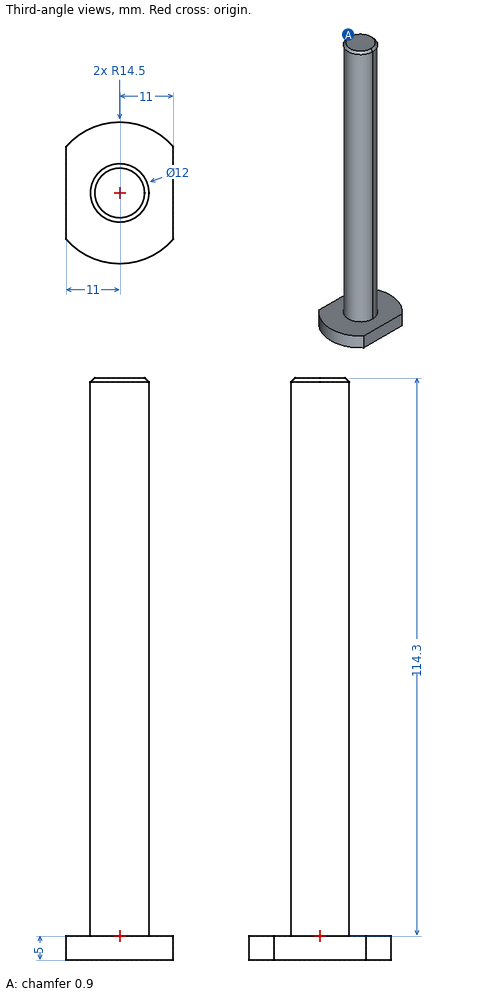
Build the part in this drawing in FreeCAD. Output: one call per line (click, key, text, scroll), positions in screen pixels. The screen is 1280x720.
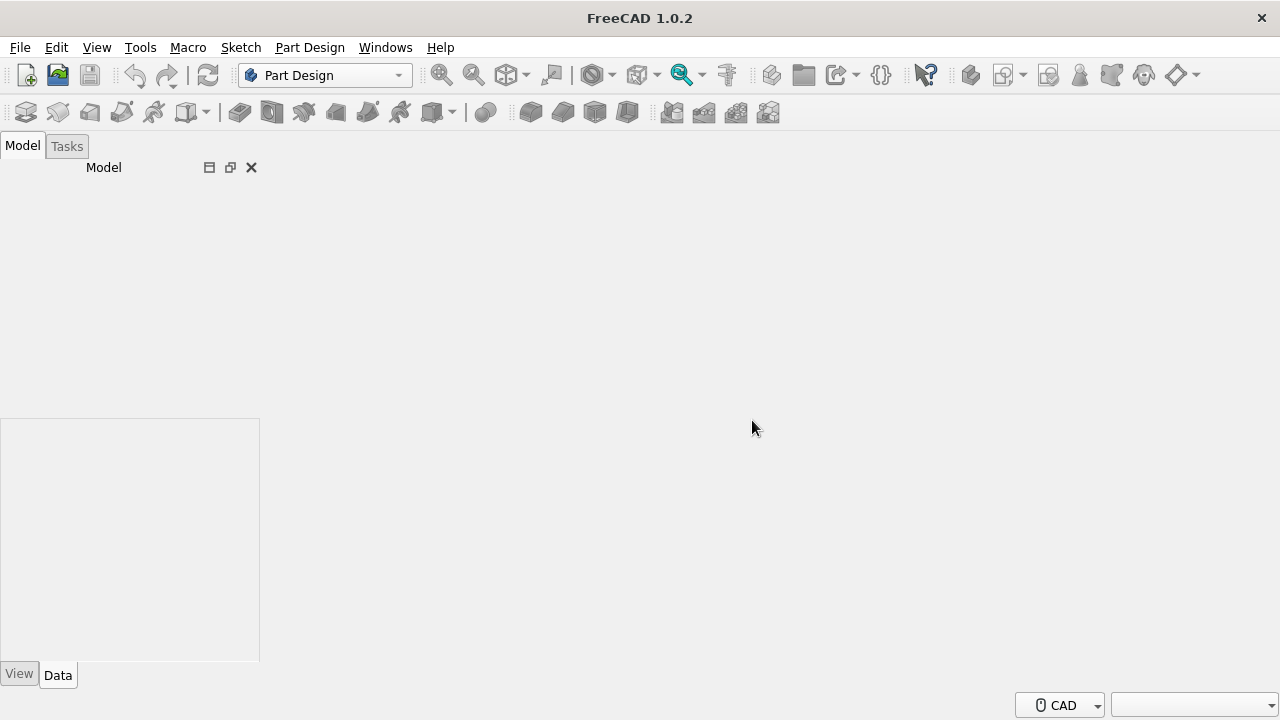
click(26, 76)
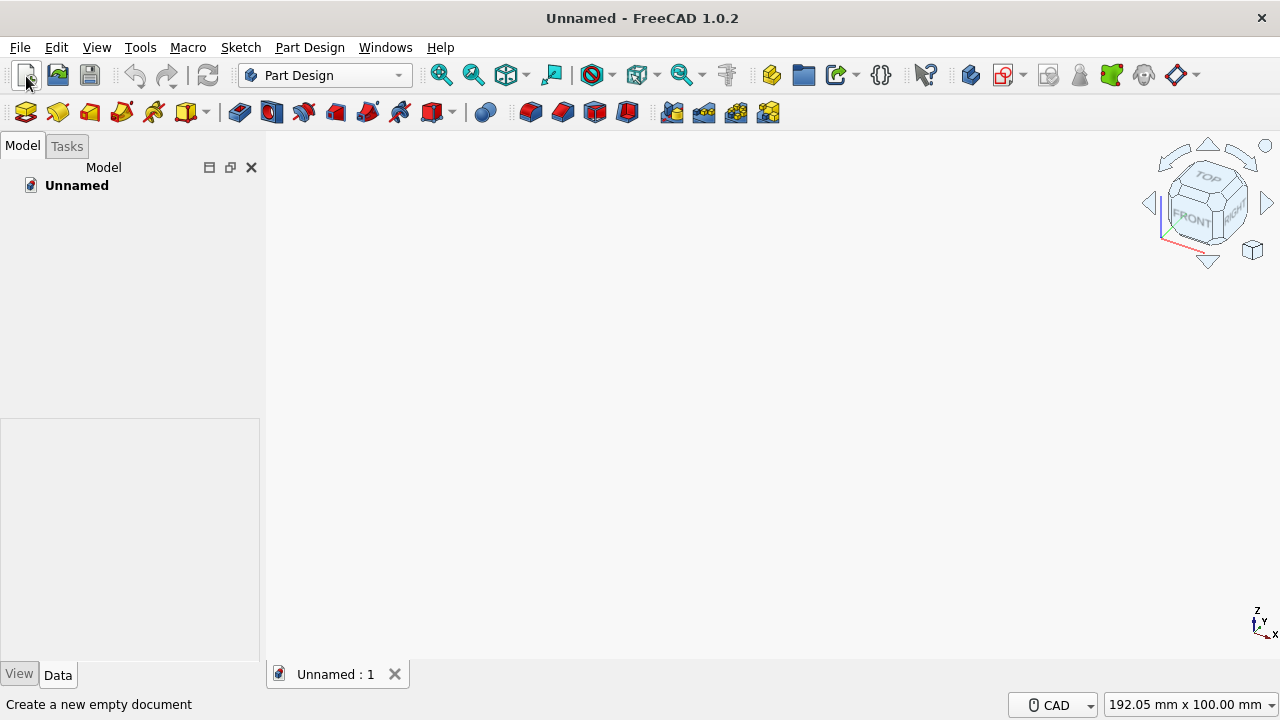
click(1004, 76)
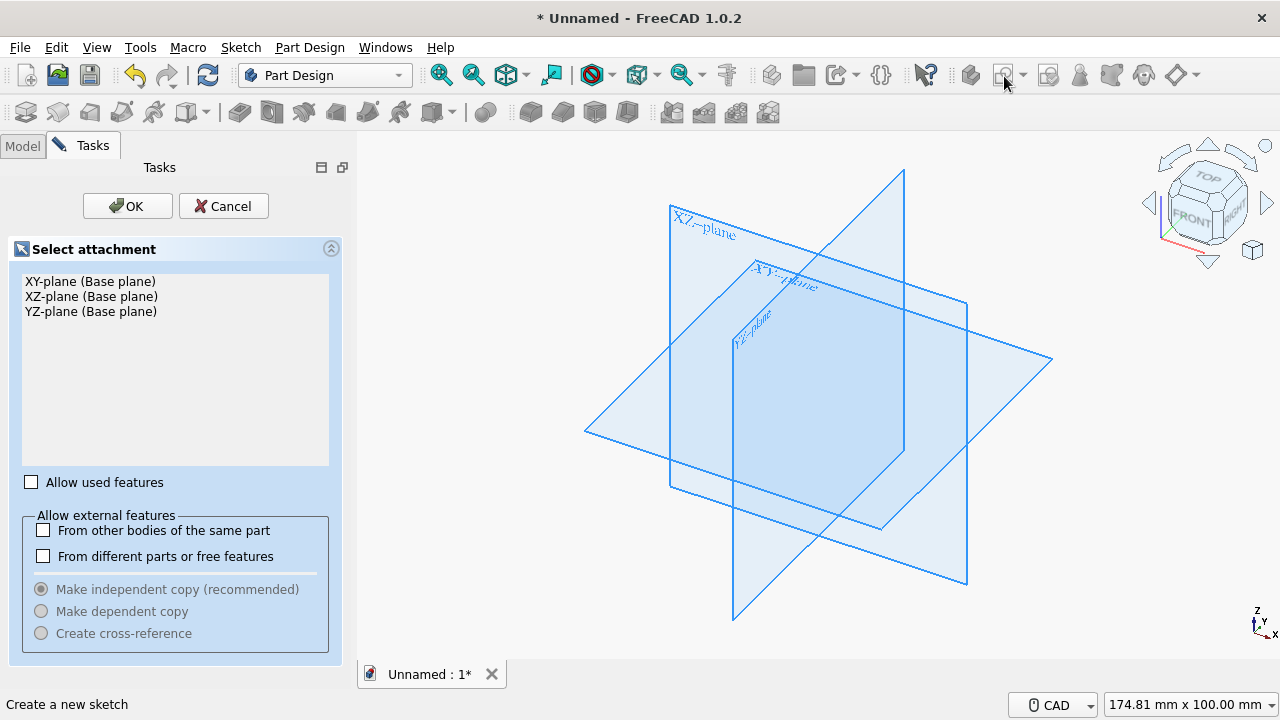
click(82, 282)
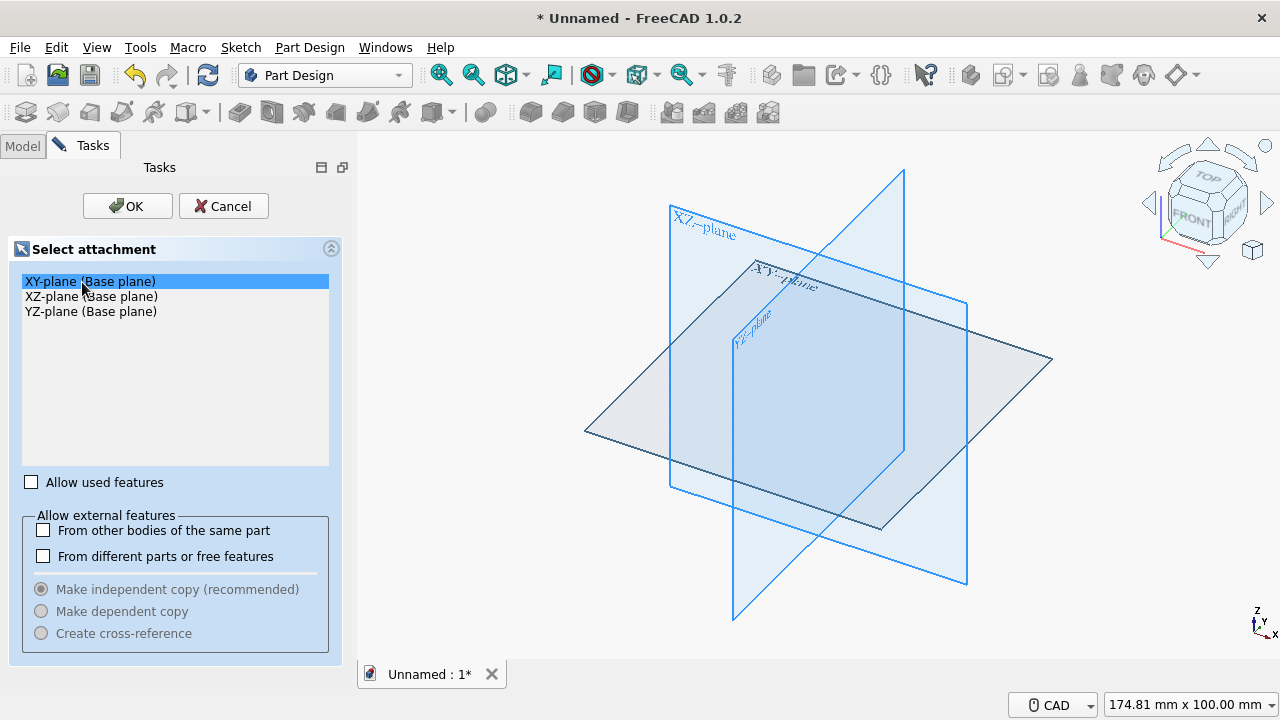
click(128, 206)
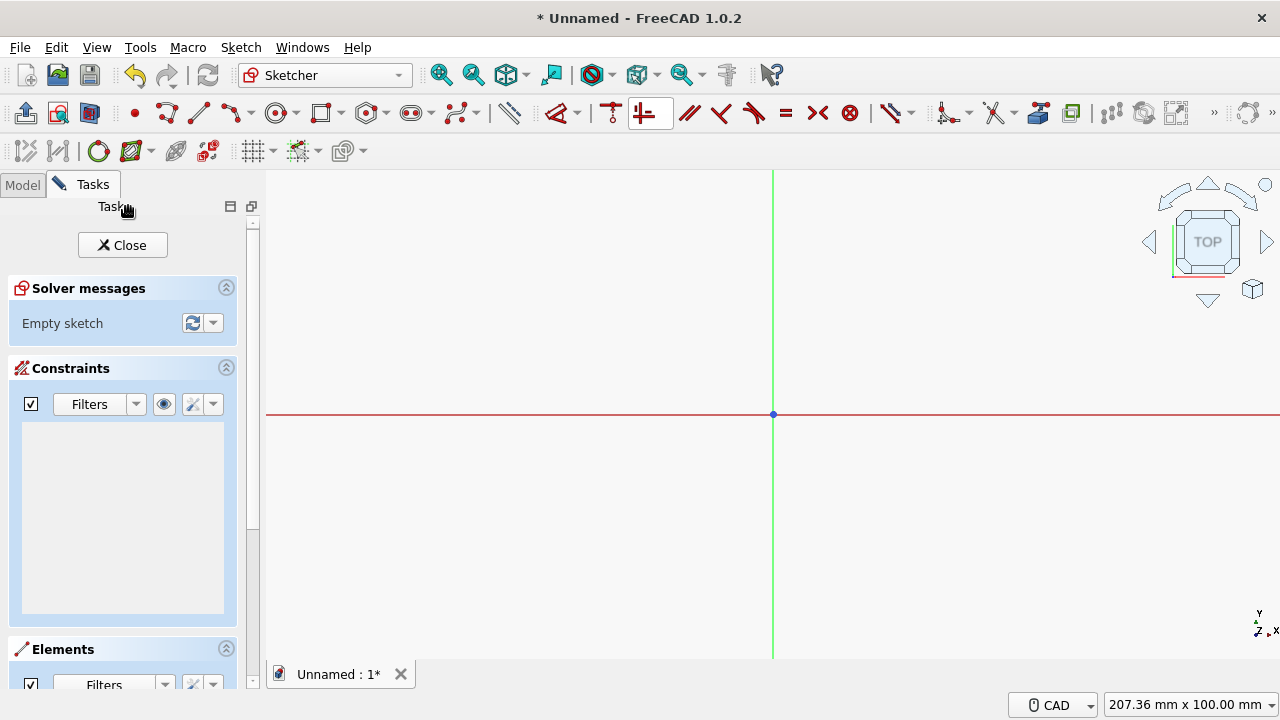
scroll(790, 414, up, 8)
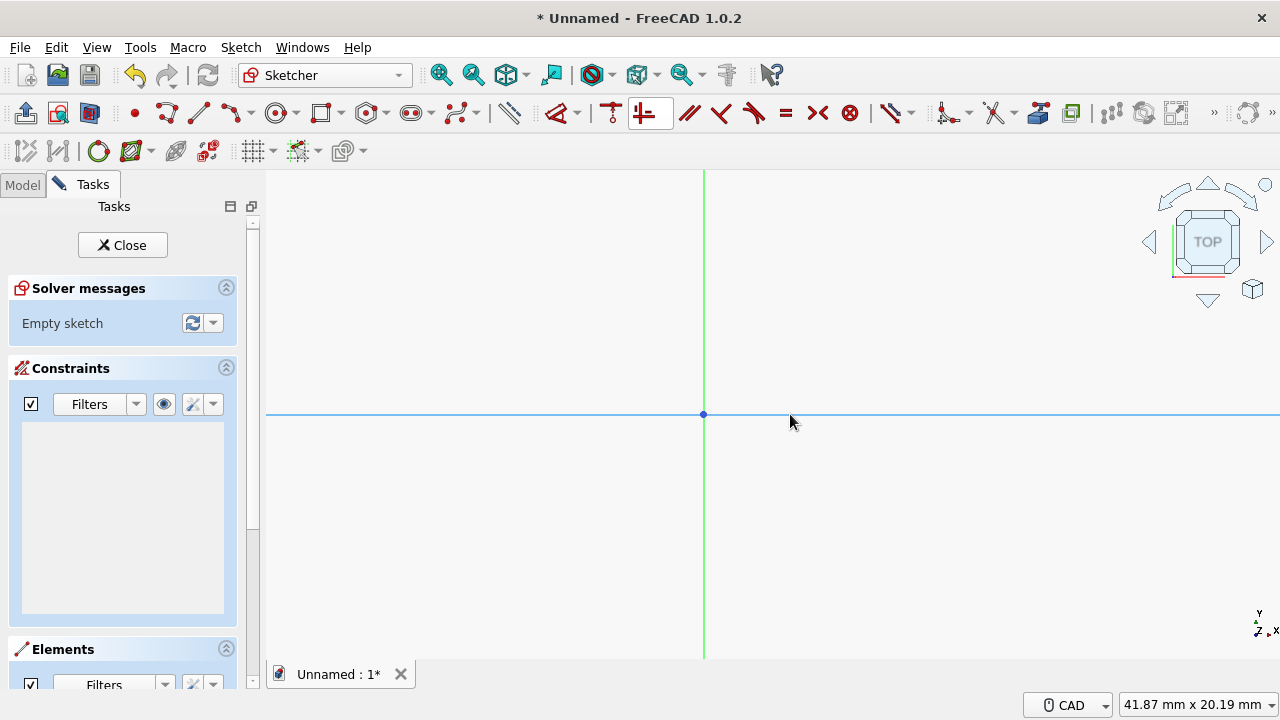
click(276, 114)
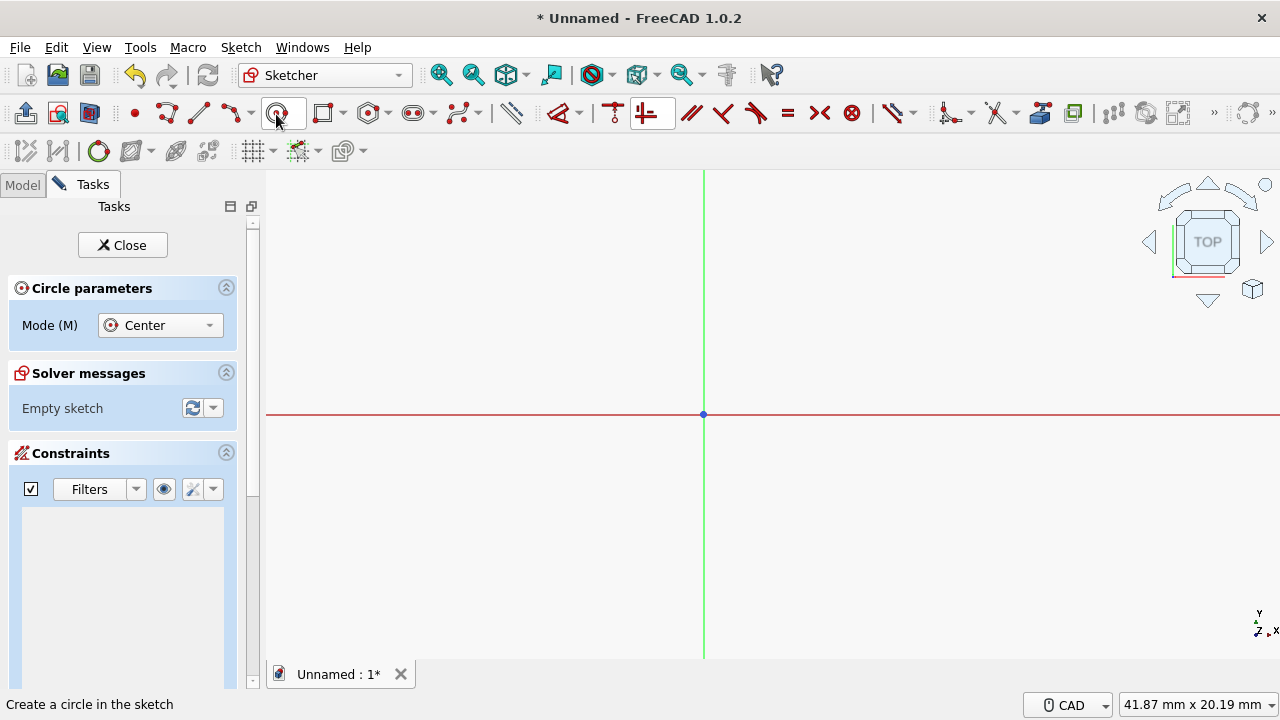
click(704, 414)
move(807, 312)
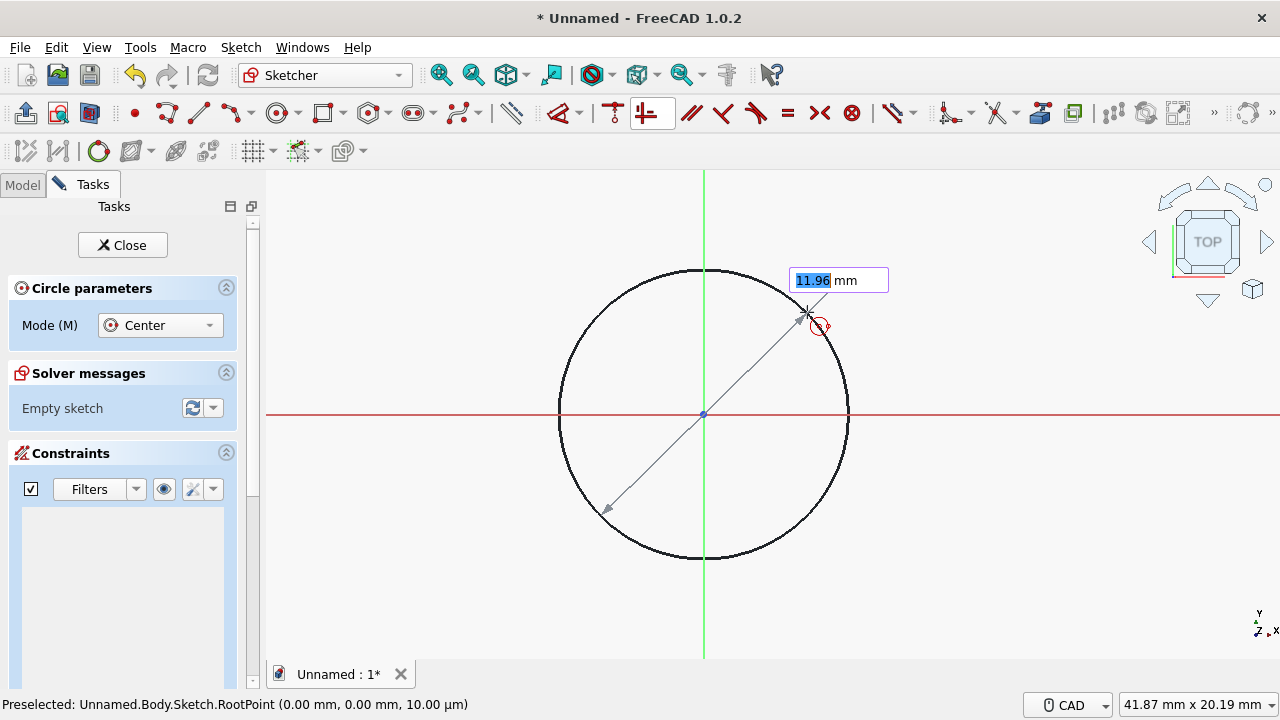
text(12)
key(Return)
key(Escape)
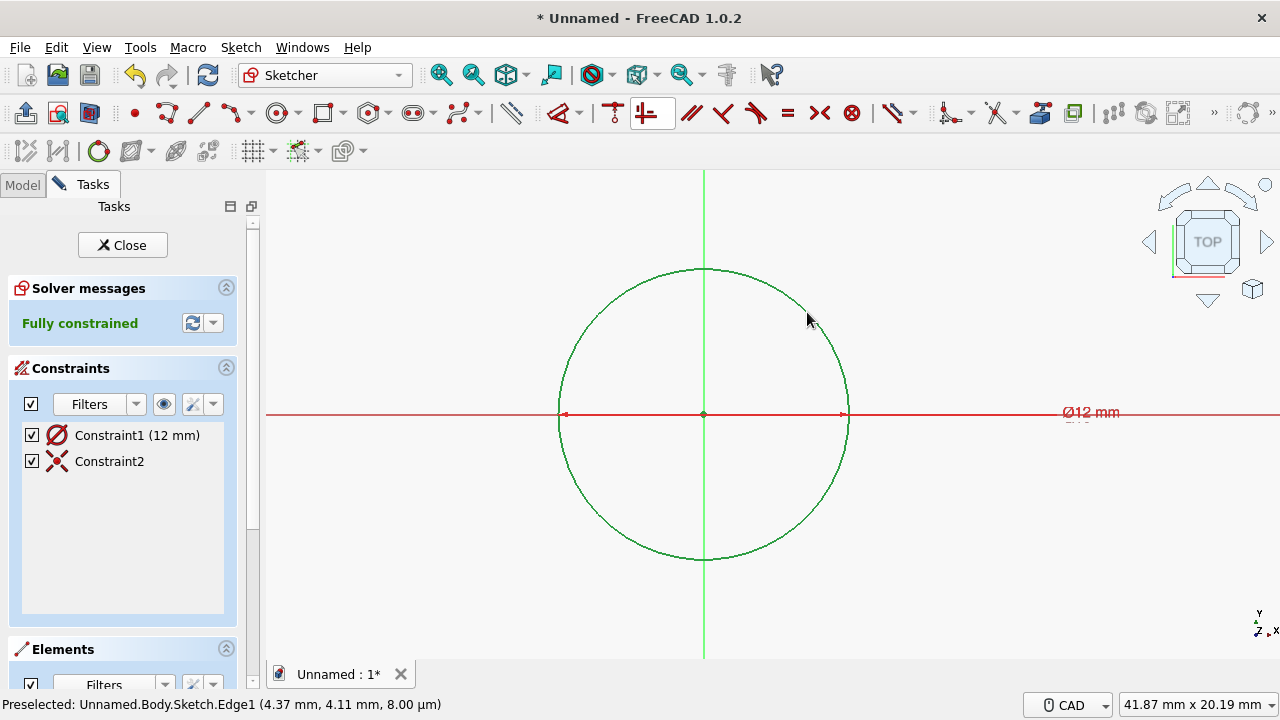
click(123, 245)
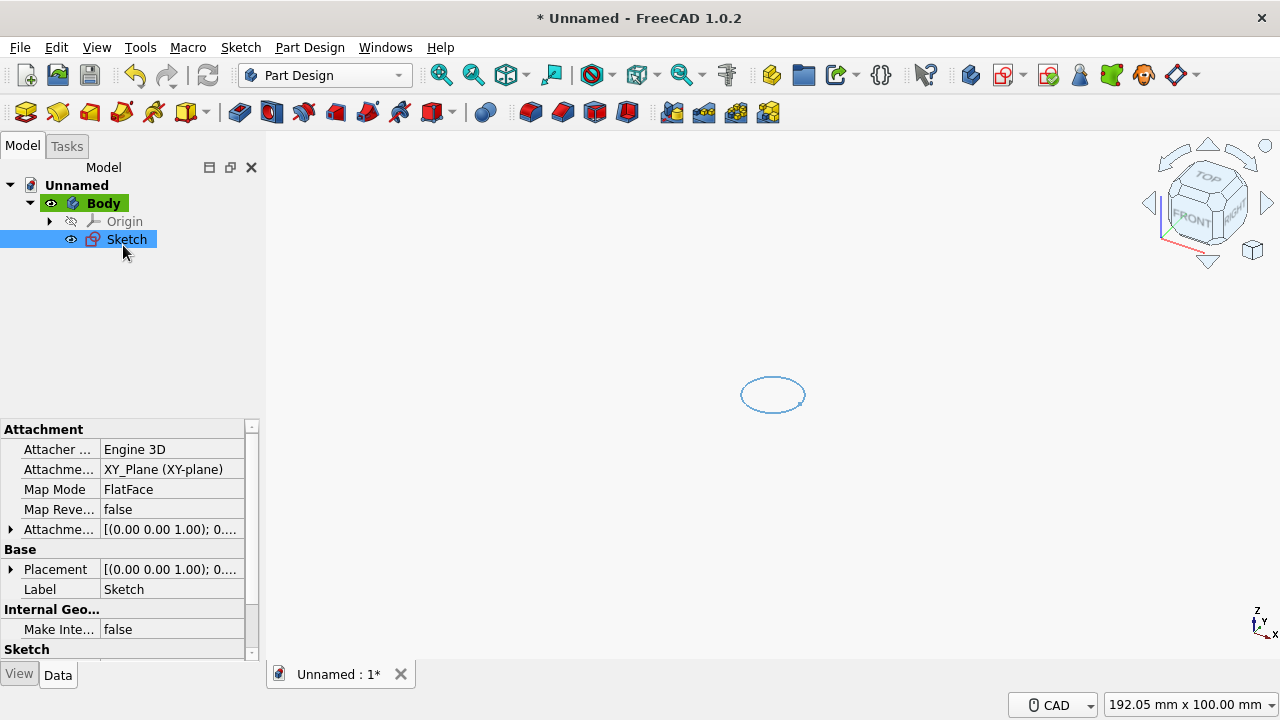
click(26, 112)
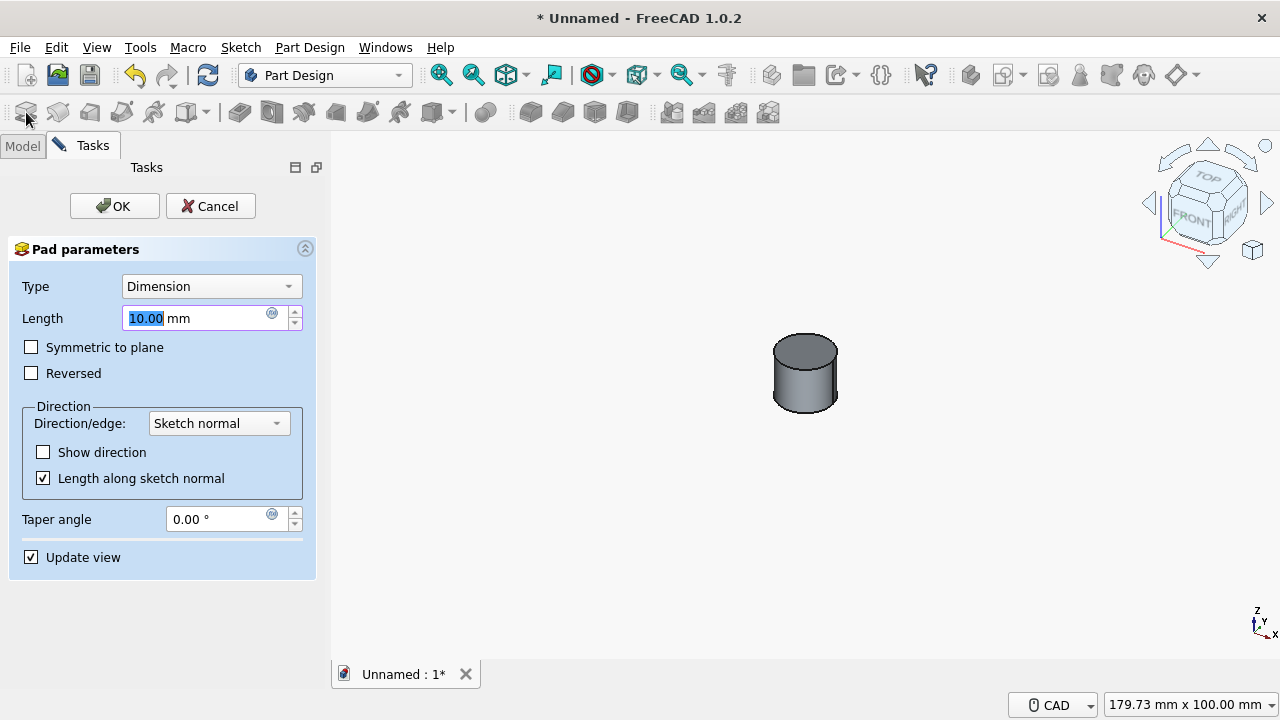
text(114.3)
key(Tab)